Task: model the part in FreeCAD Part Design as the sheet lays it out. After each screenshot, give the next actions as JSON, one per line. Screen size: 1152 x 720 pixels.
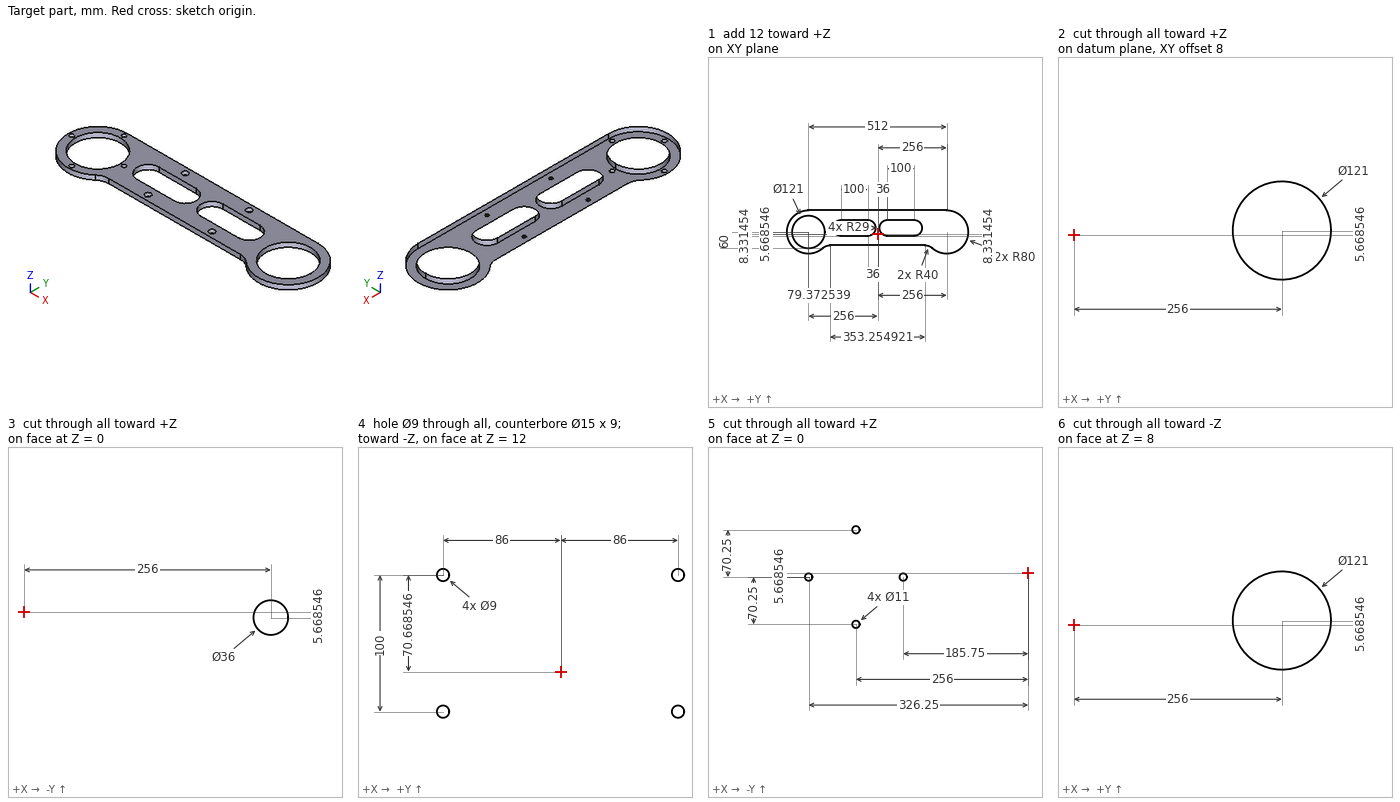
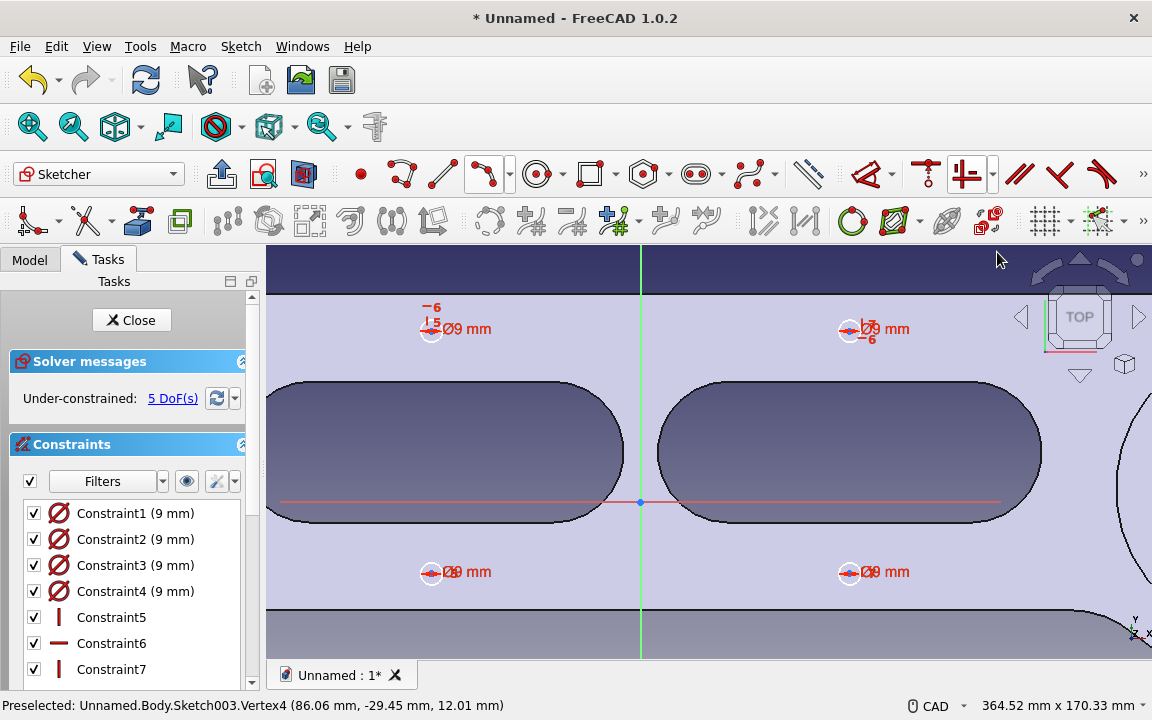
{"action": "left_click", "coordinate": [432, 574]}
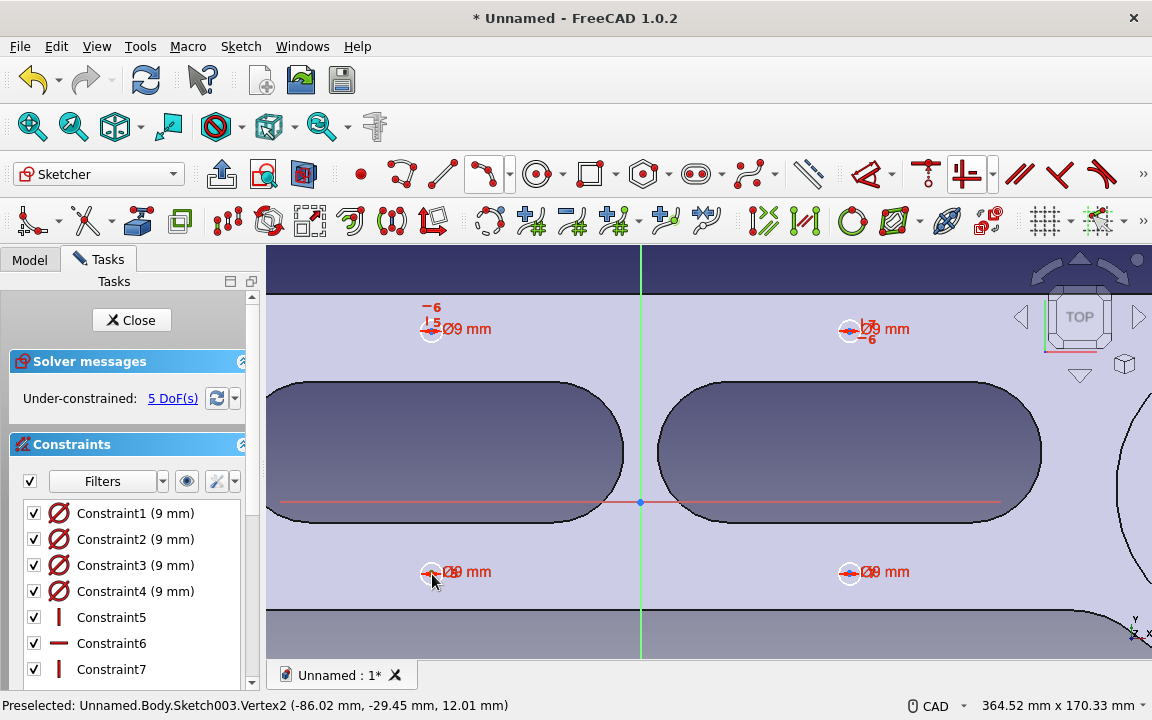
{"action": "left_click", "coordinate": [850, 574]}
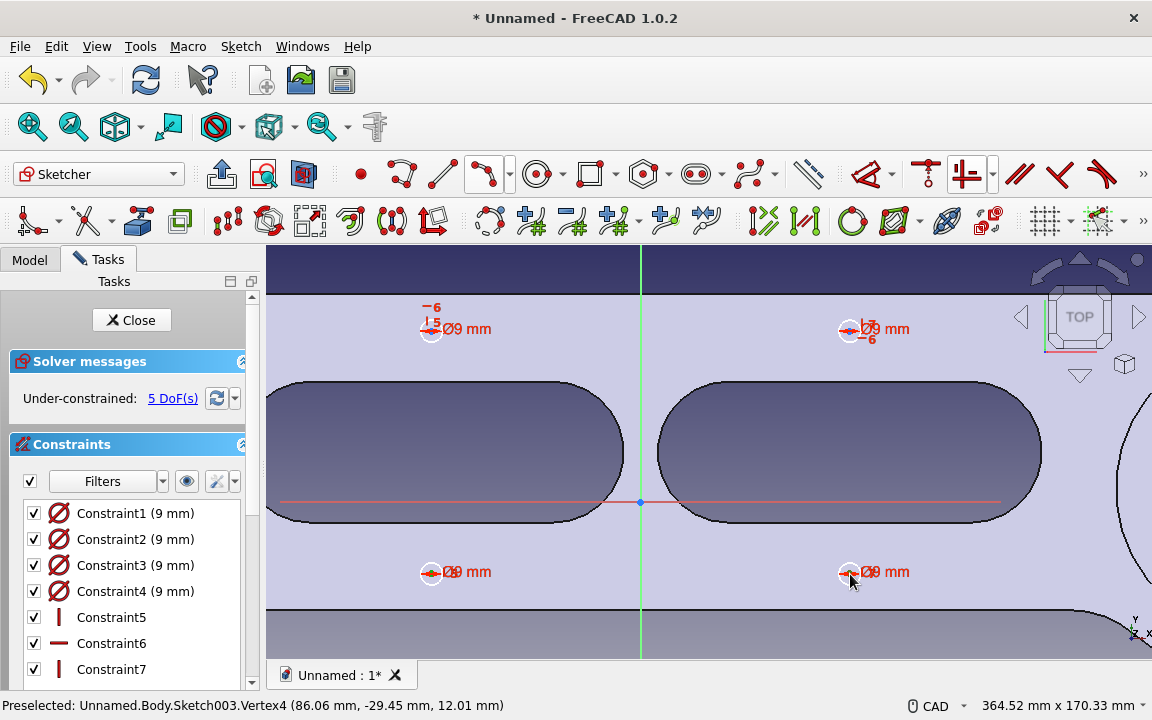
{"action": "key", "text": "h"}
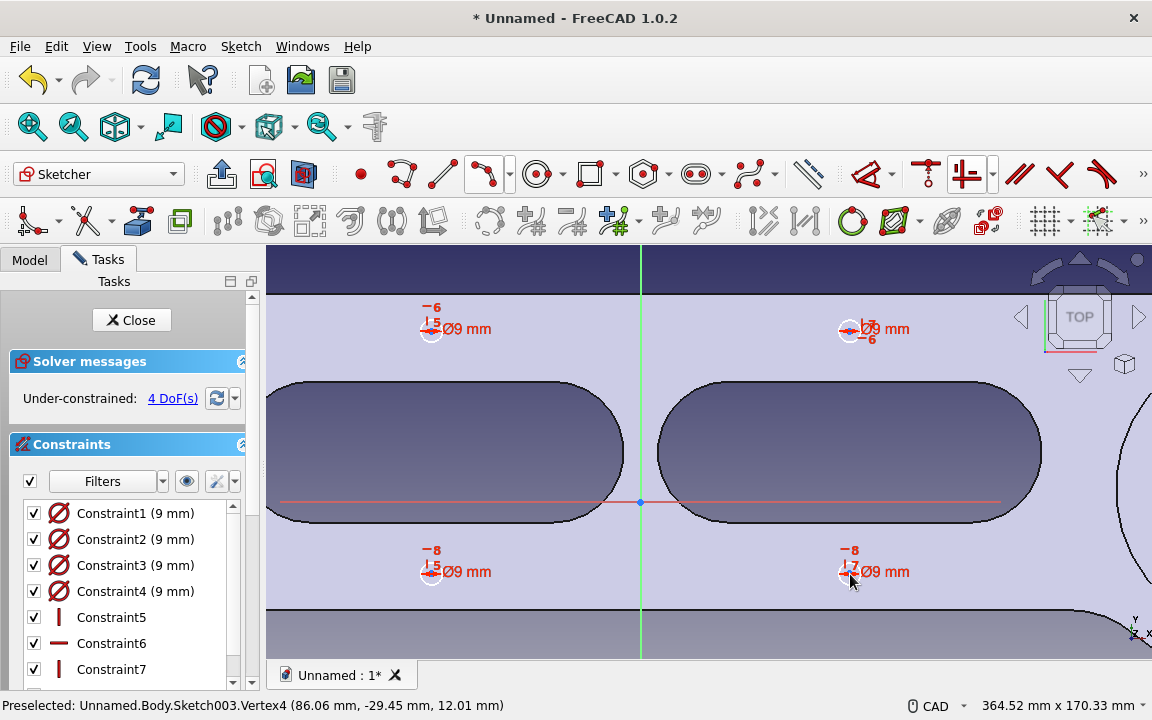
{"action": "left_click", "coordinate": [866, 174]}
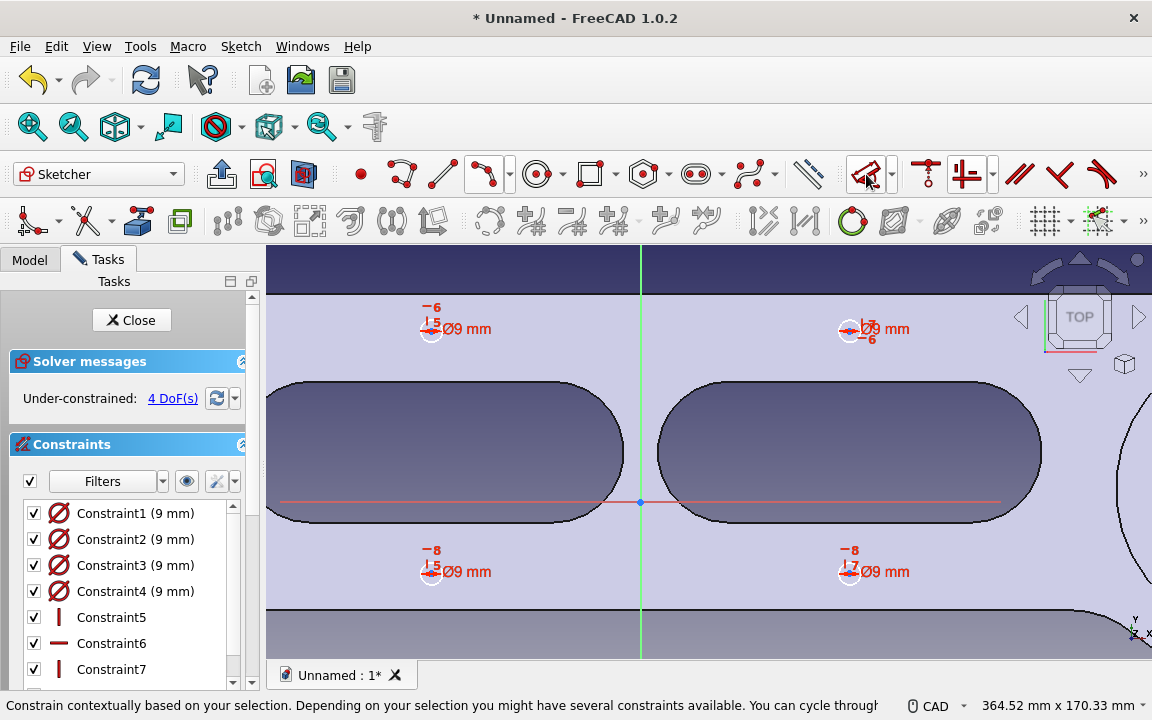
{"action": "left_click", "coordinate": [432, 331]}
{"action": "left_click", "coordinate": [536, 297]}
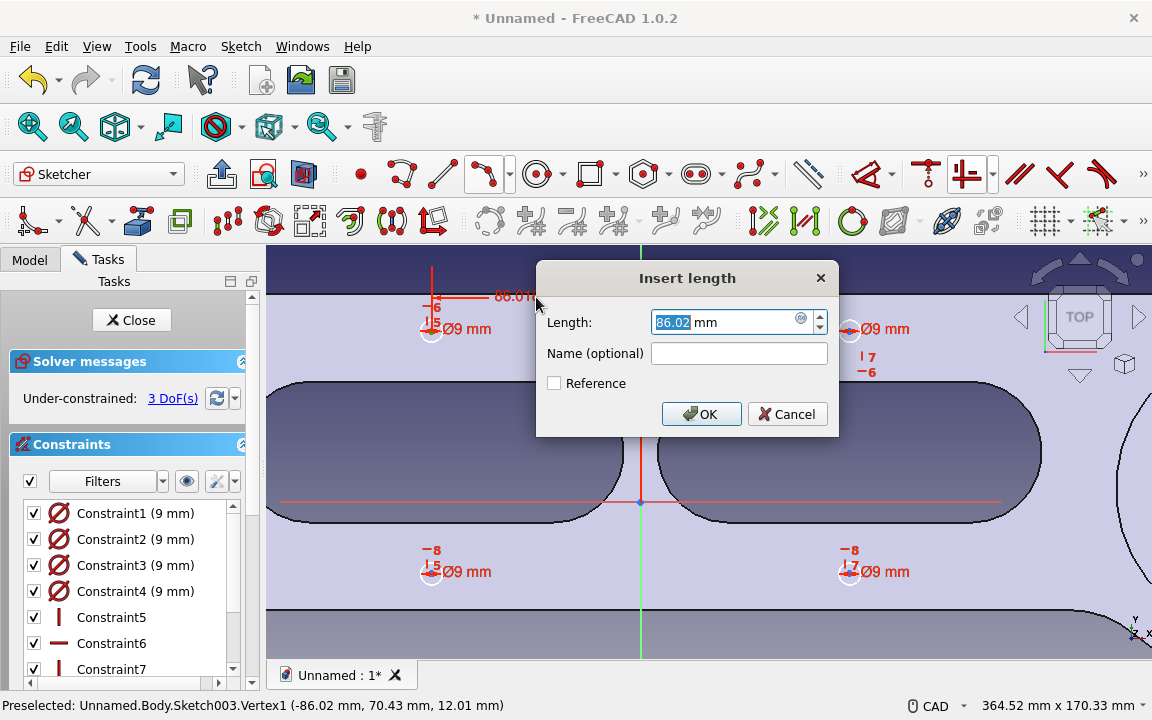
{"action": "type", "text": "86"}
{"action": "key", "text": "Return"}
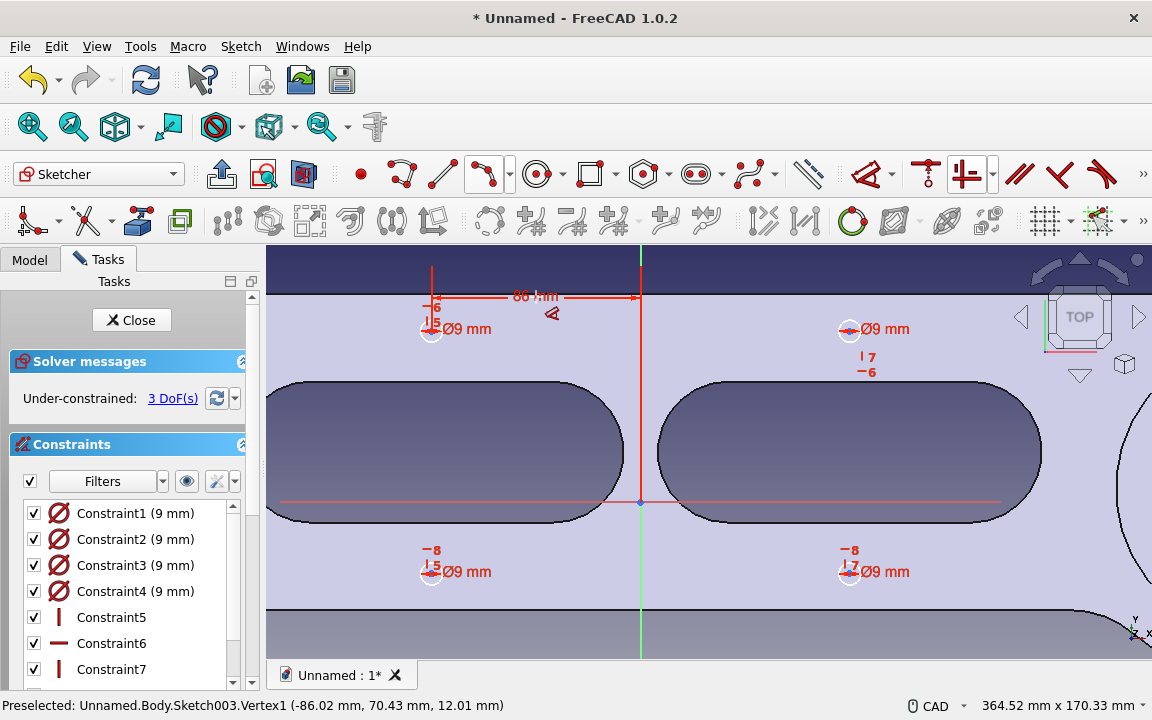
{"action": "left_click", "coordinate": [850, 331]}
{"action": "left_click", "coordinate": [745, 297]}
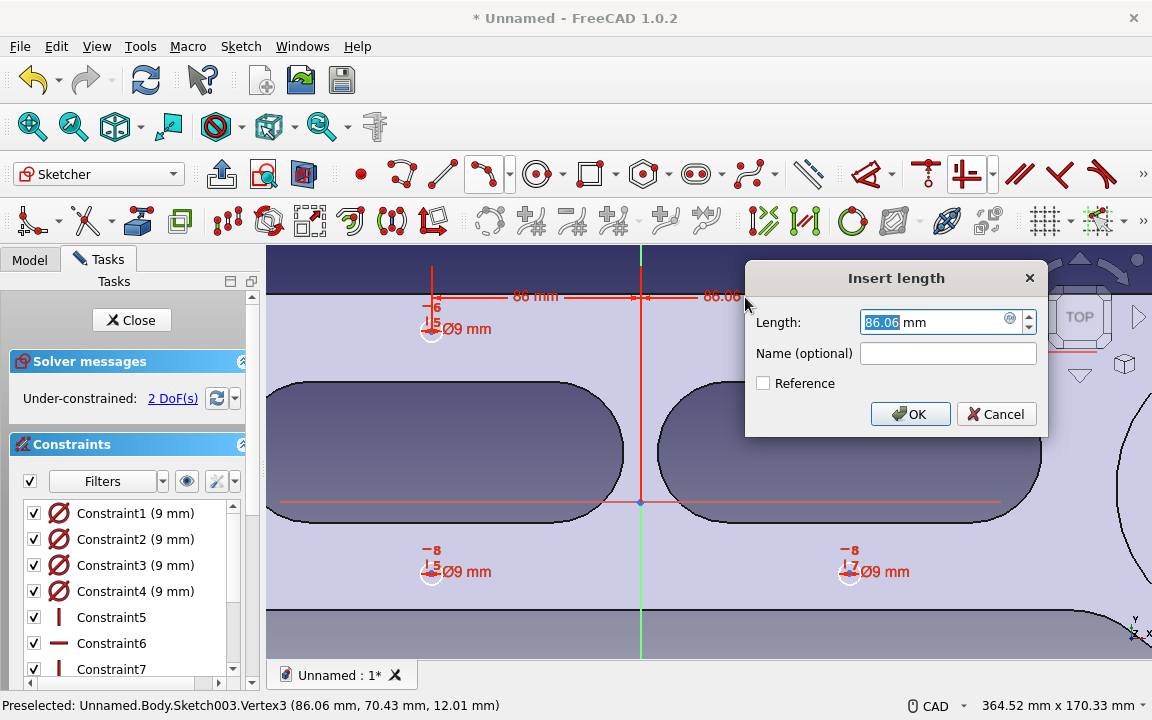
{"action": "type", "text": "86"}
{"action": "key", "text": "Return"}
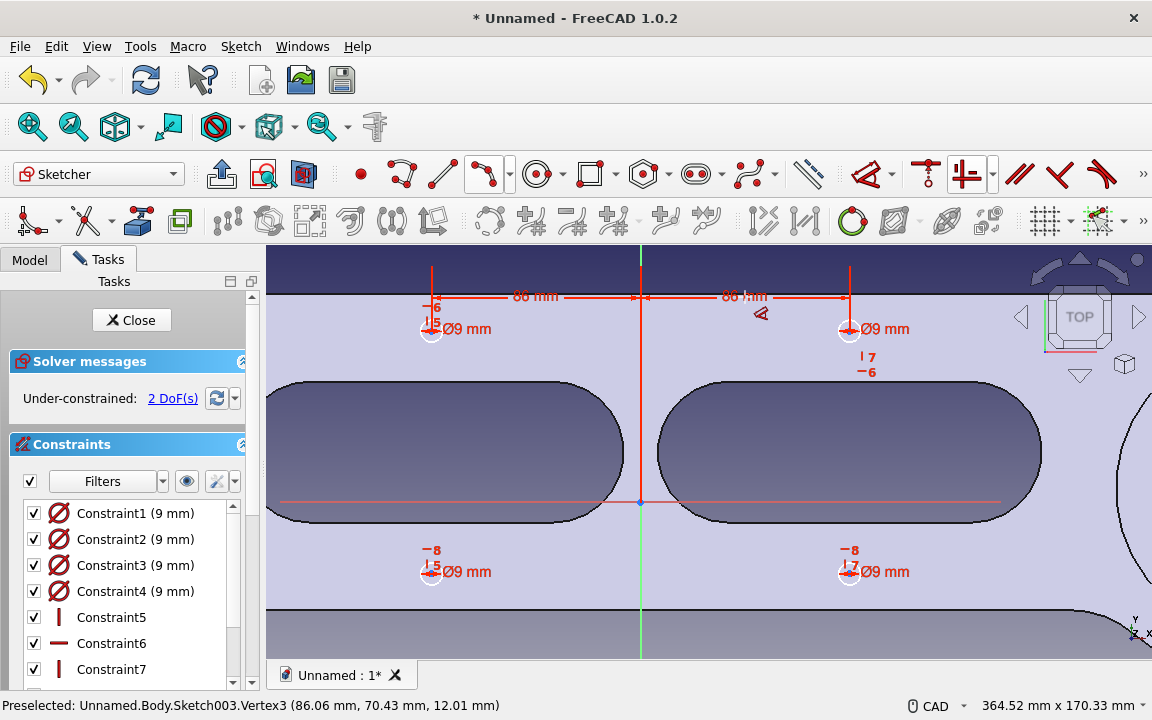
{"action": "left_click", "coordinate": [432, 331]}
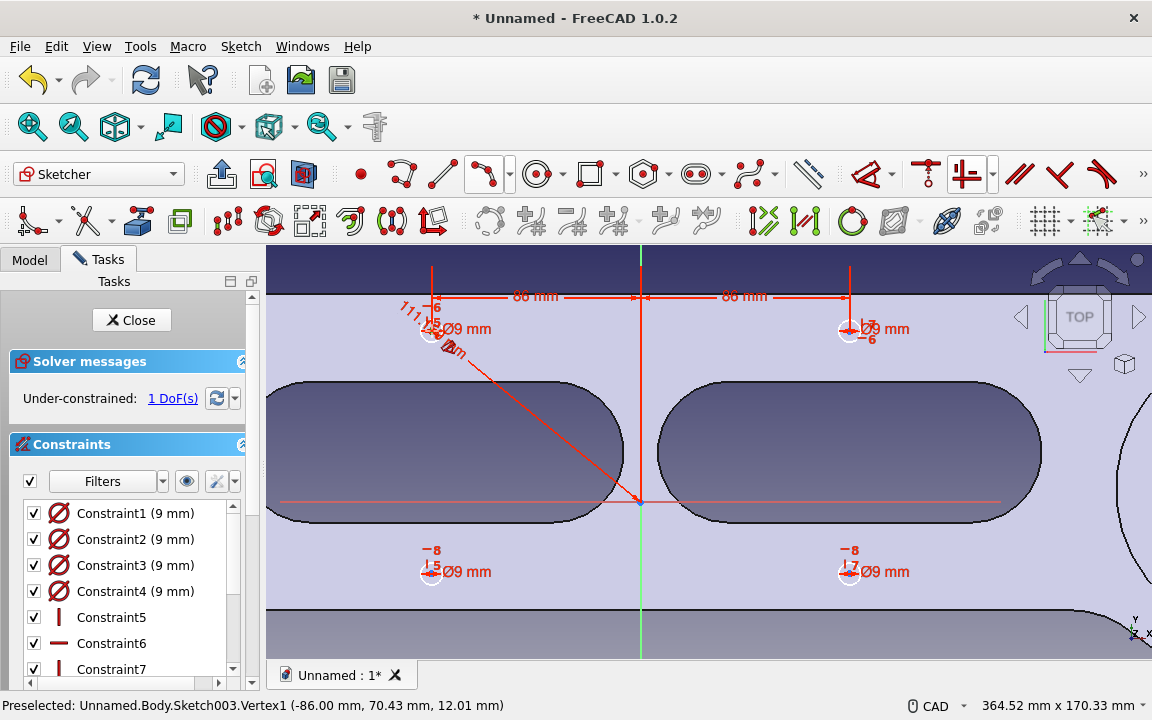
{"action": "left_click", "coordinate": [432, 574]}
{"action": "left_click", "coordinate": [398, 453]}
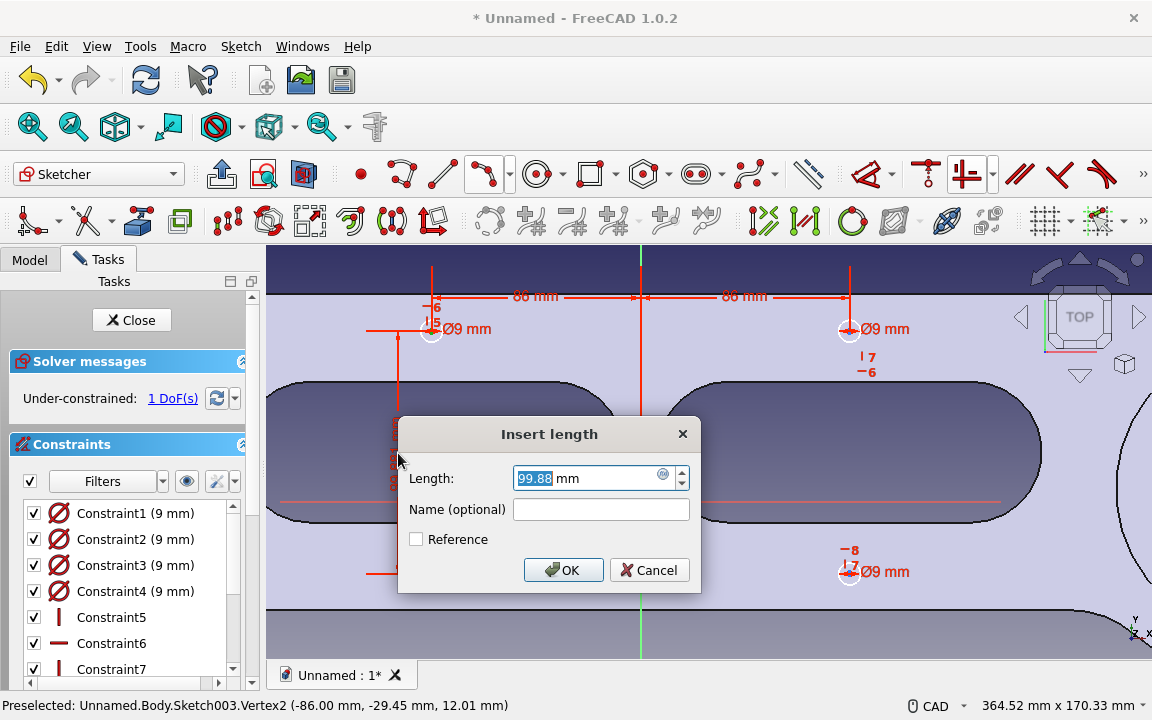
{"action": "type", "text": "100"}
{"action": "key", "text": "Return"}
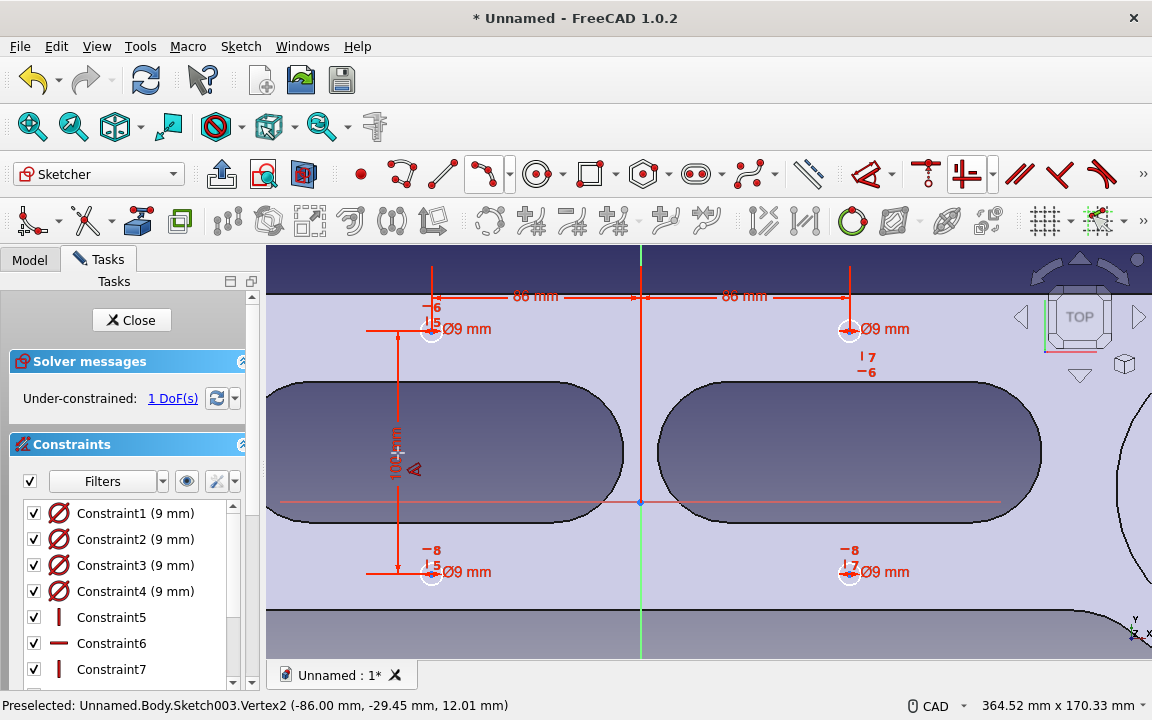
{"action": "left_click", "coordinate": [432, 331]}
{"action": "left_click", "coordinate": [398, 417]}